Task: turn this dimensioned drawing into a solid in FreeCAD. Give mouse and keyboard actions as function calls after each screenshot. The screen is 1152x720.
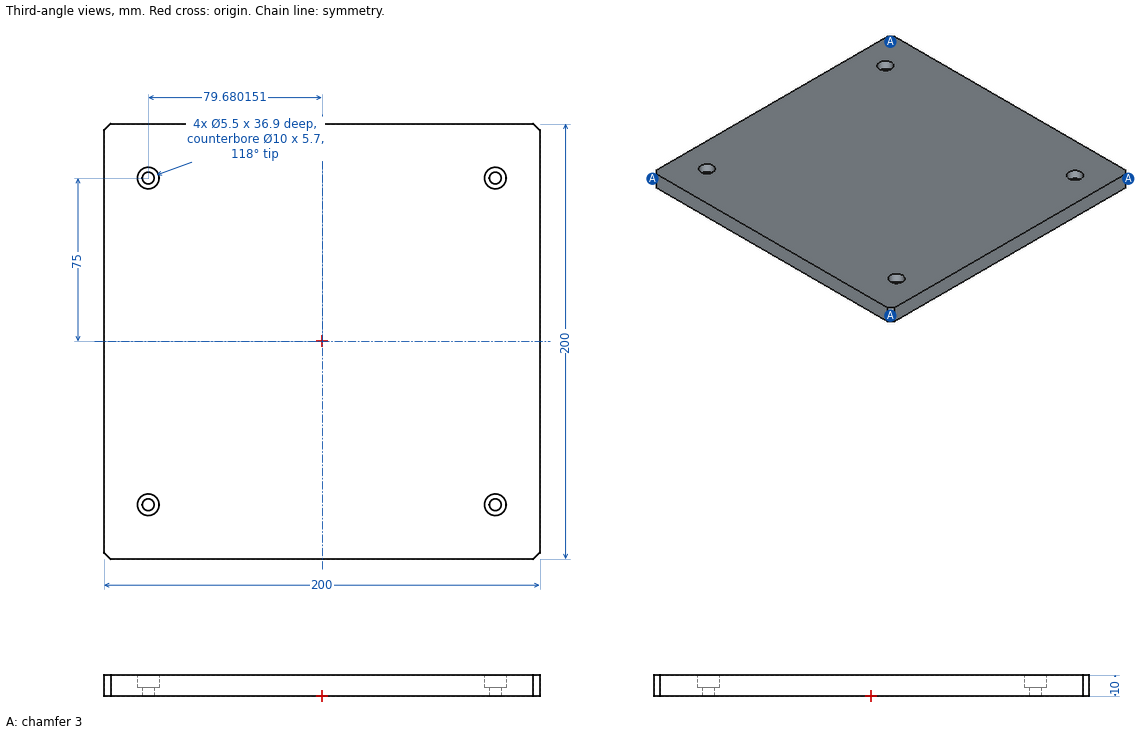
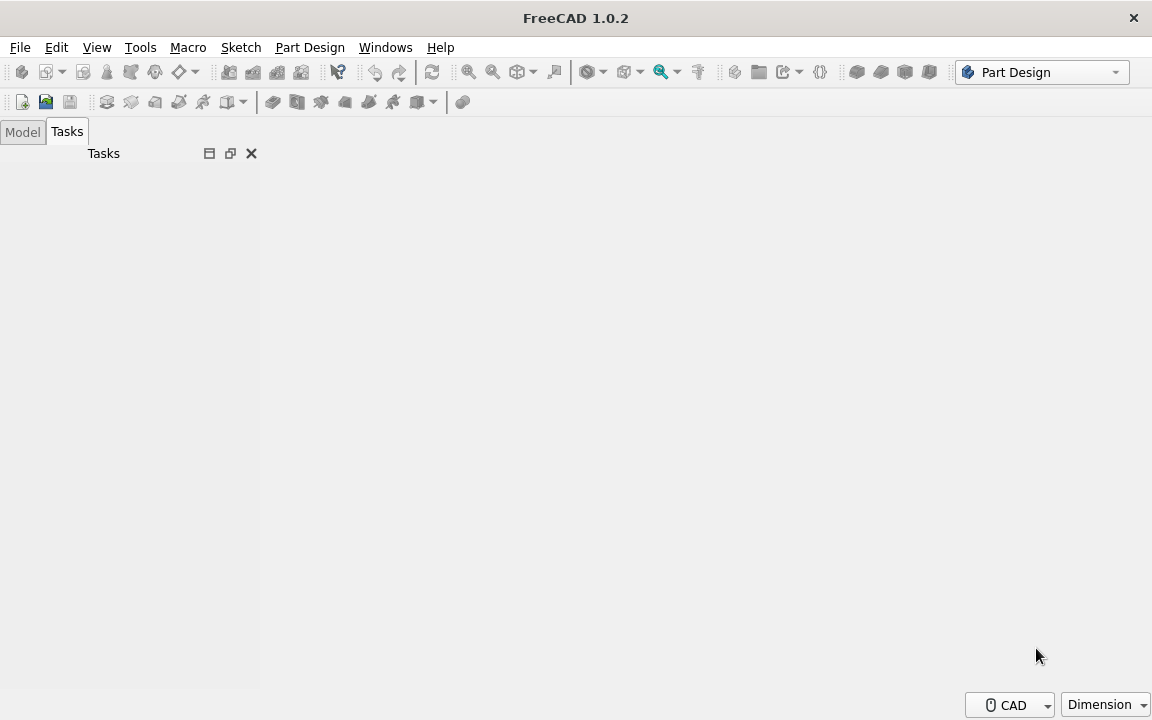
key(ctrl+n)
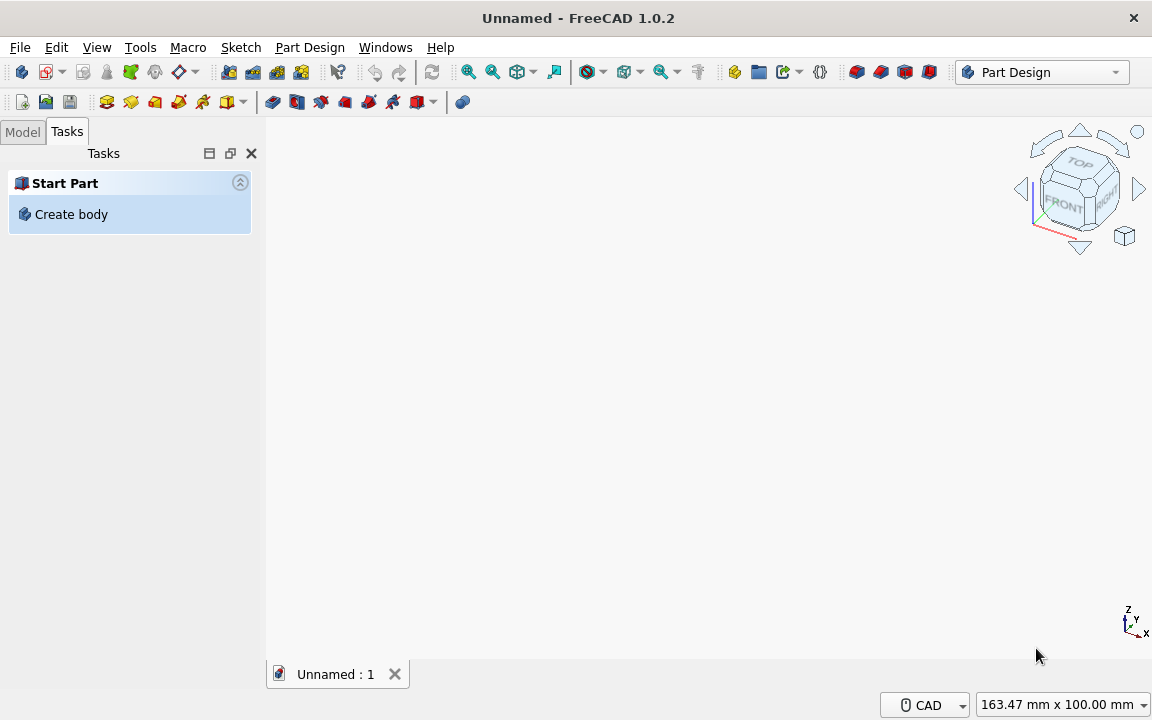
click(46, 72)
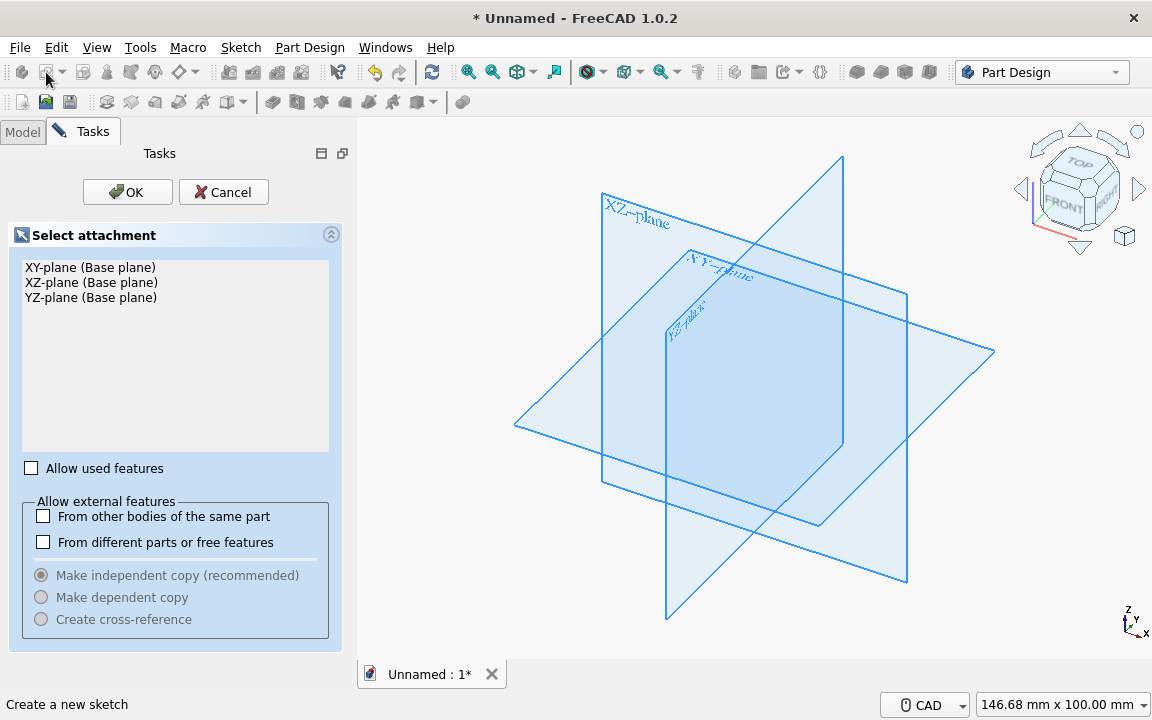
click(82, 268)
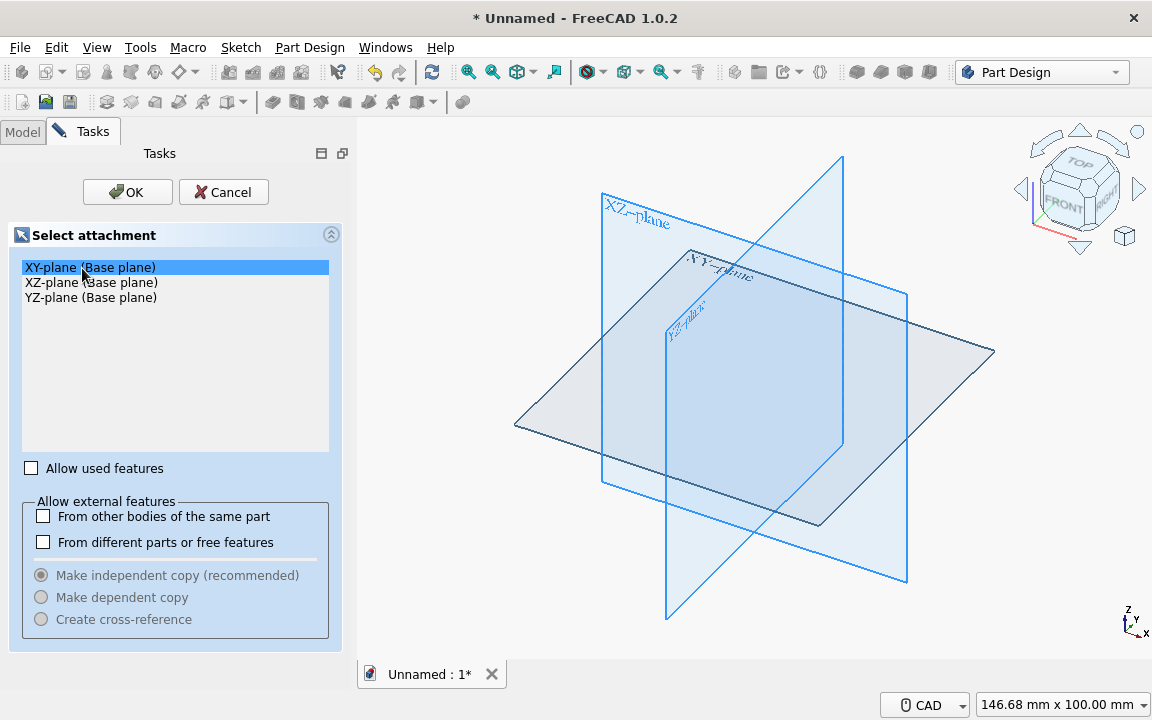
click(128, 192)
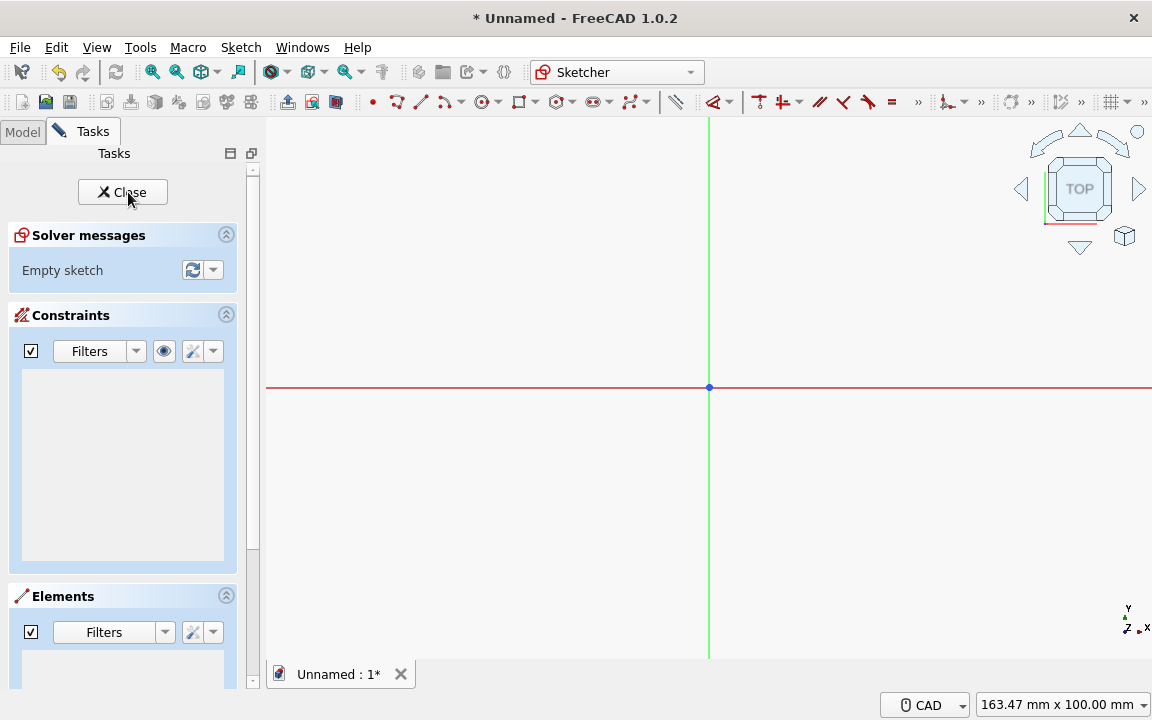
scroll(611, 388, down, 6)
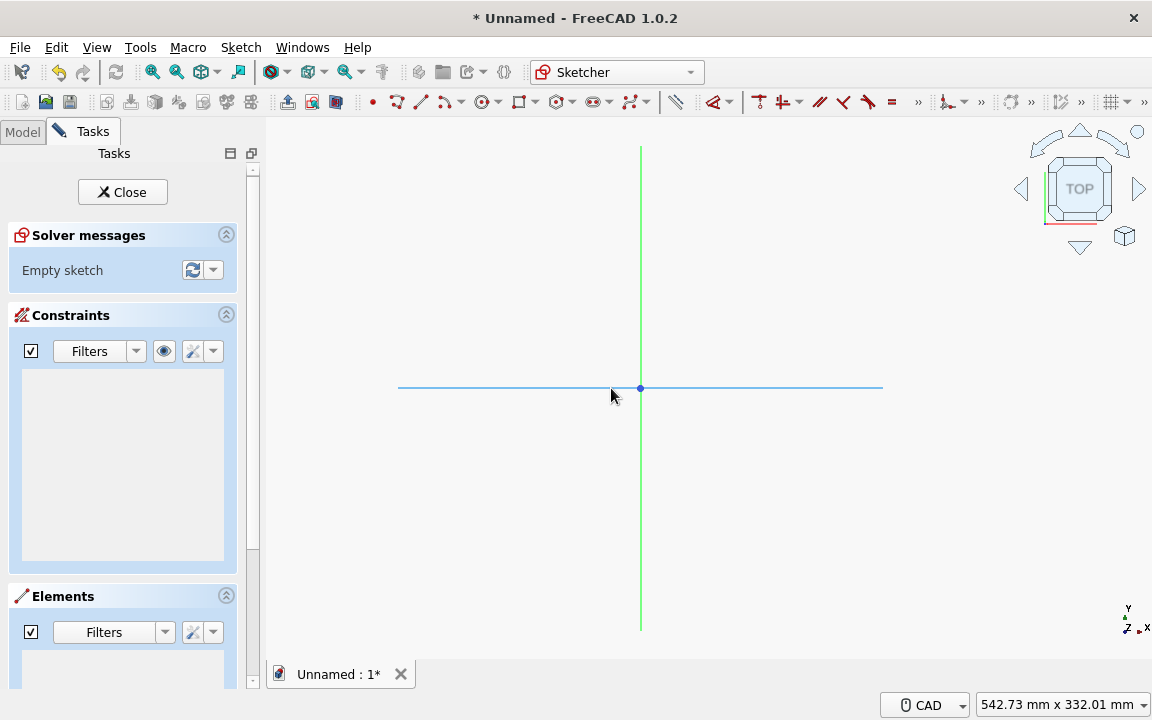
click(538, 102)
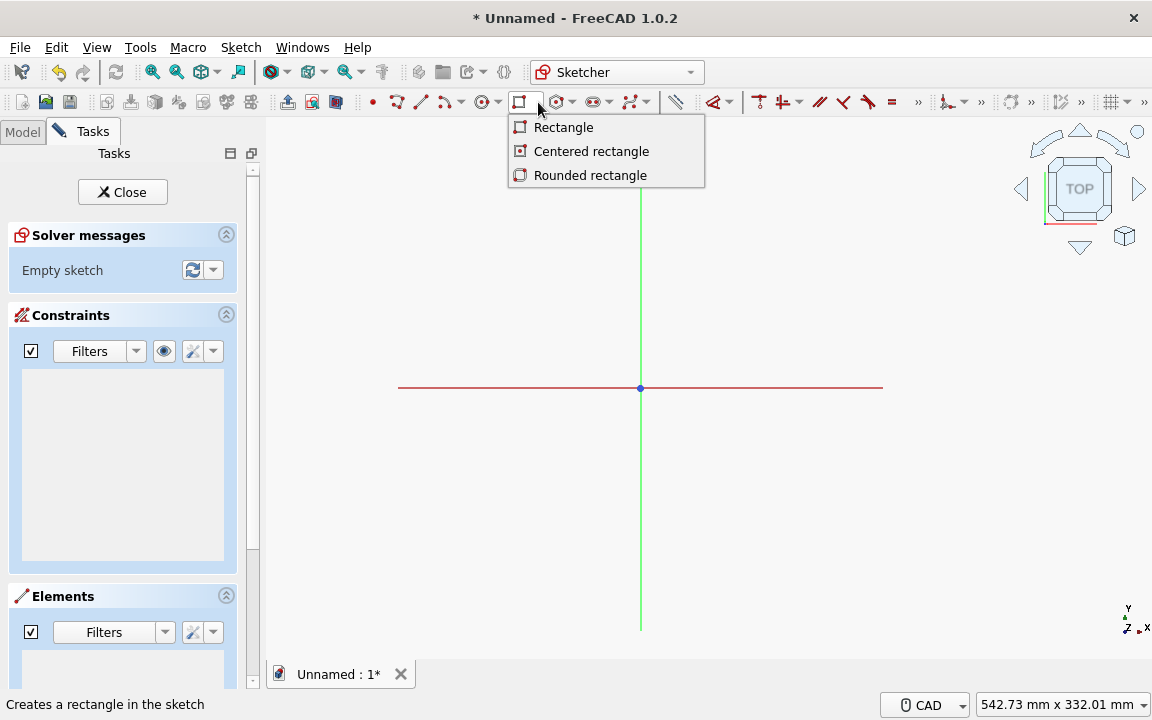
click(606, 151)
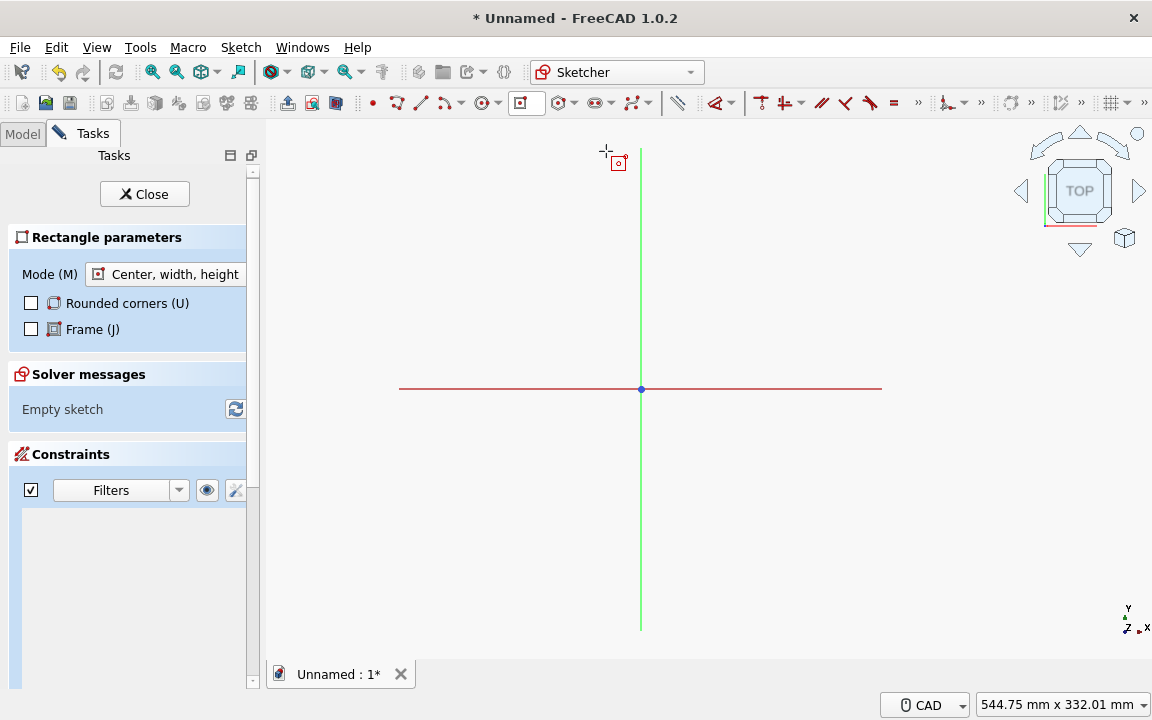
click(641, 389)
move(804, 227)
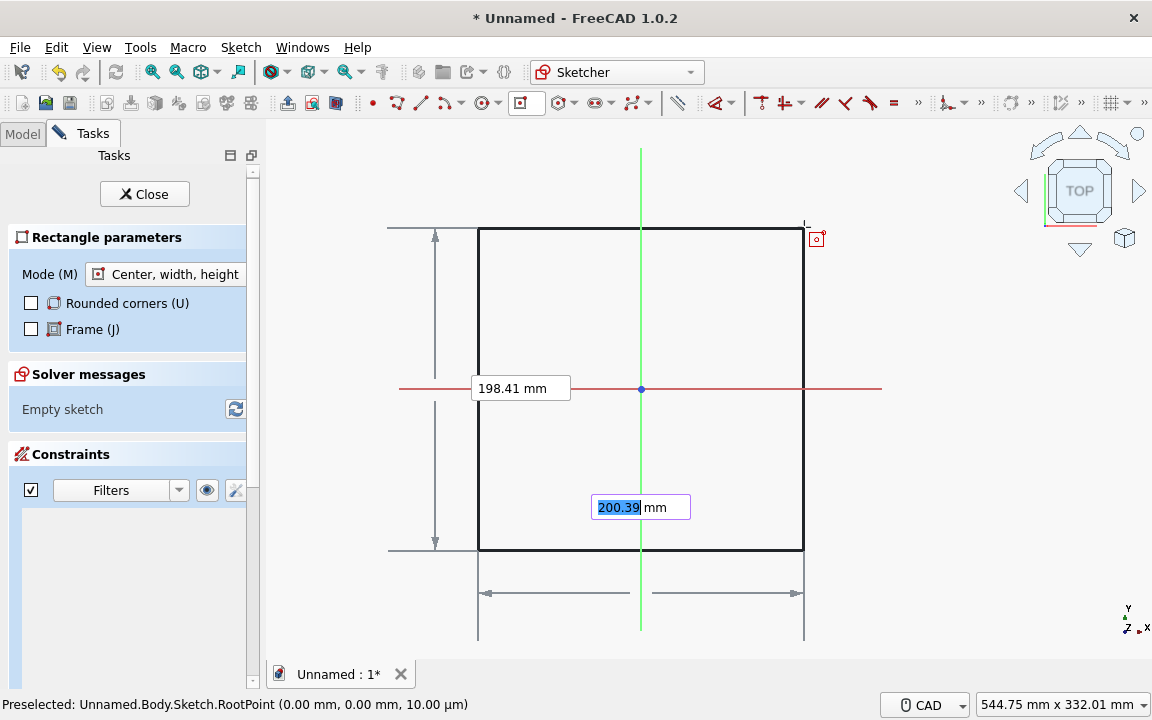
text(200)
key(Tab)
text(200)
key(Return)
key(Escape)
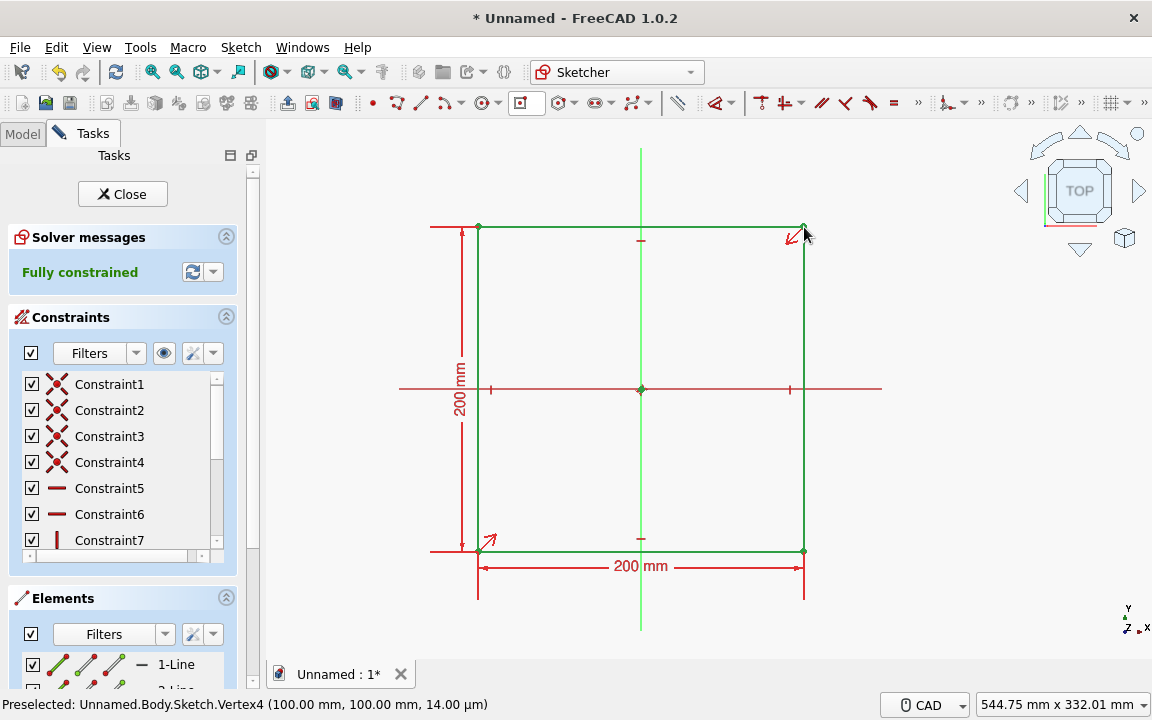
click(123, 194)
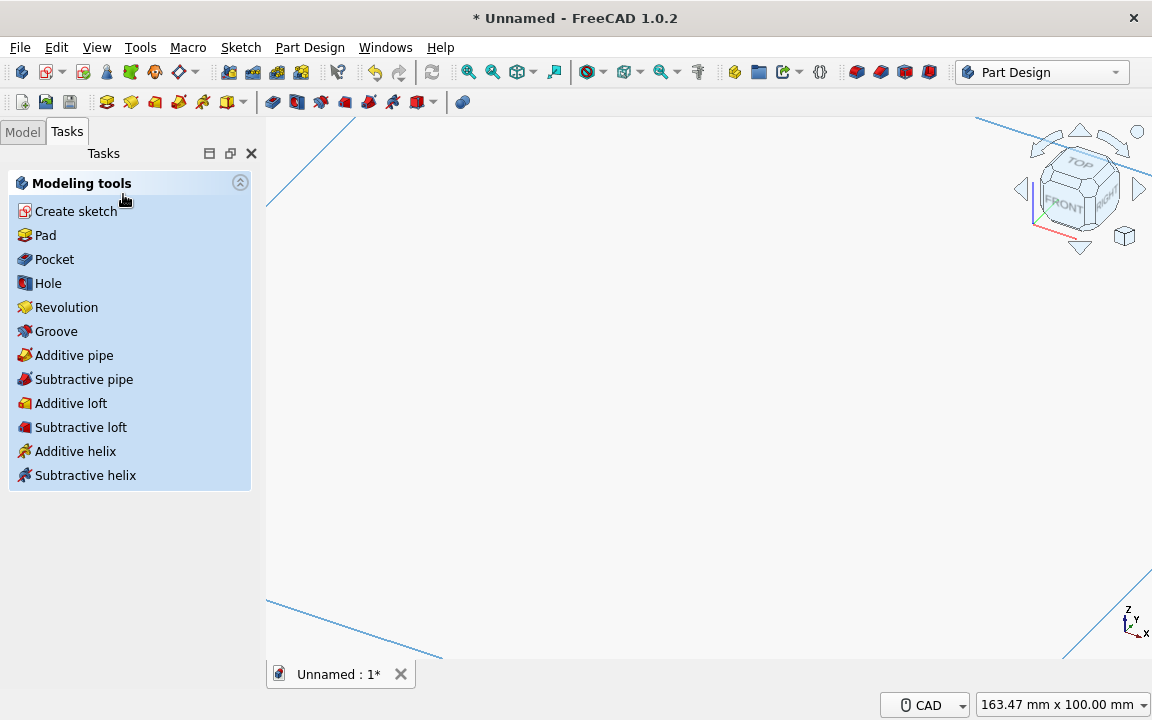
click(108, 102)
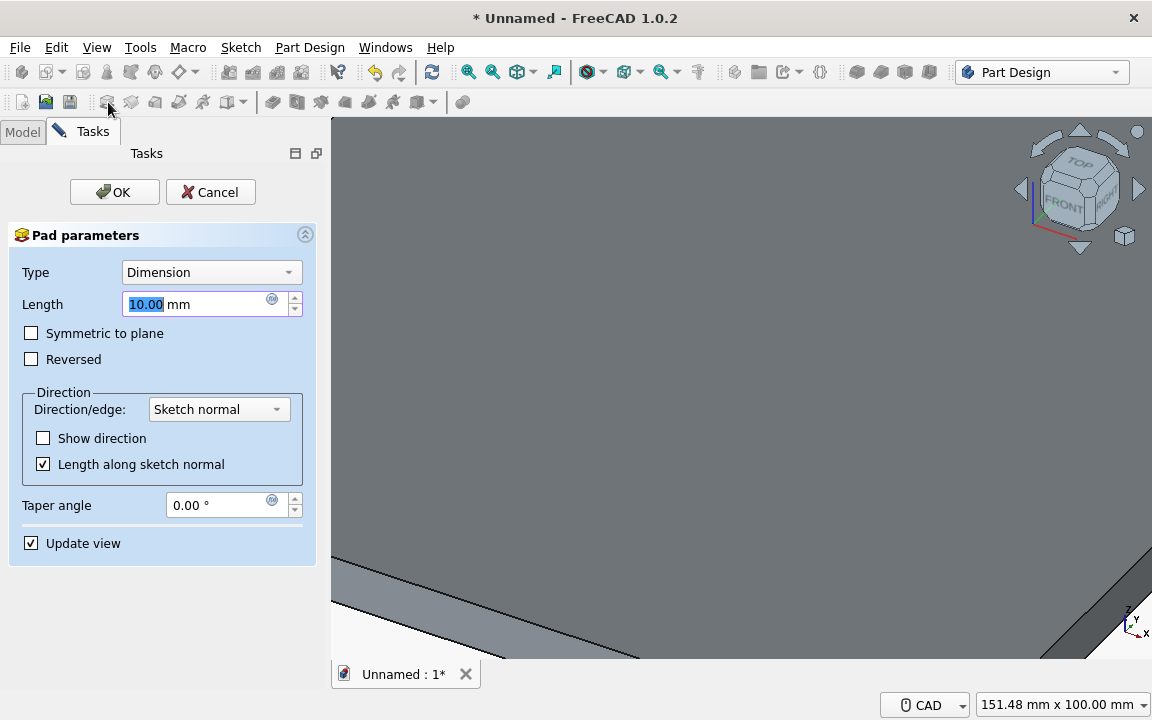
text(10)
key(Tab)